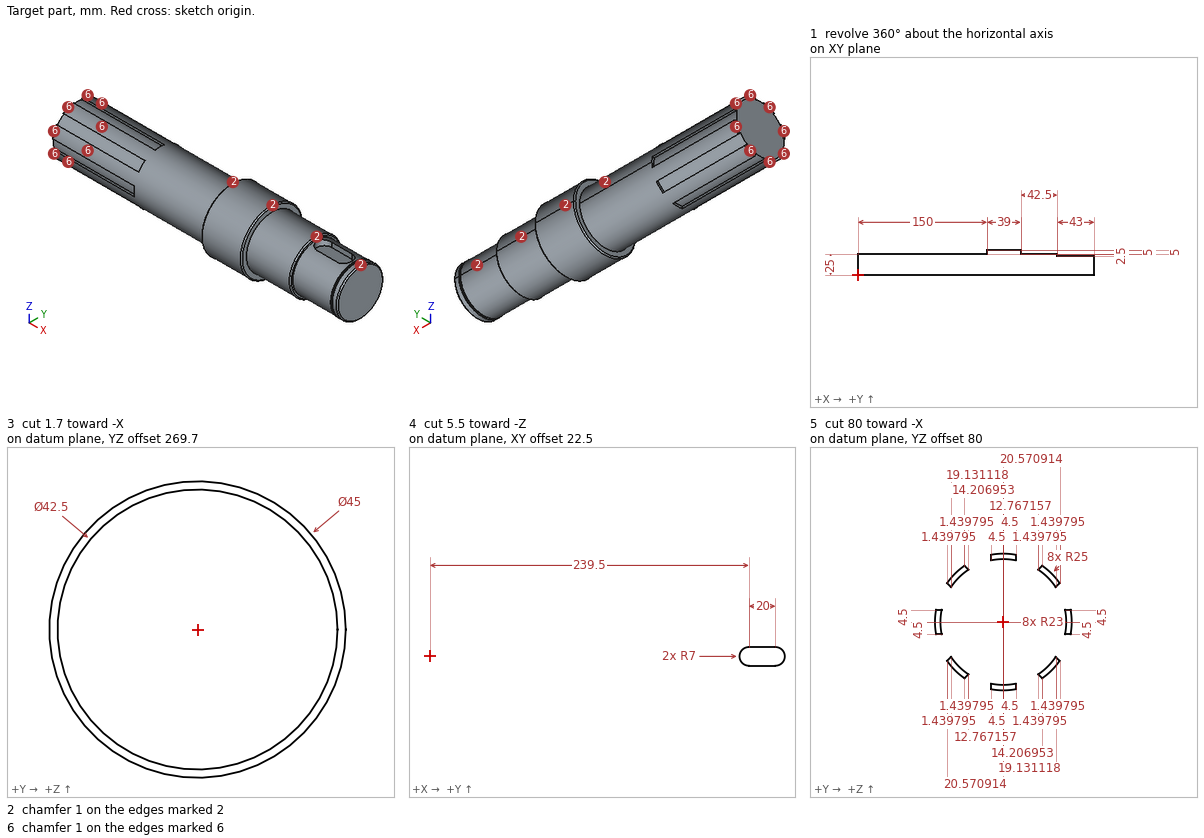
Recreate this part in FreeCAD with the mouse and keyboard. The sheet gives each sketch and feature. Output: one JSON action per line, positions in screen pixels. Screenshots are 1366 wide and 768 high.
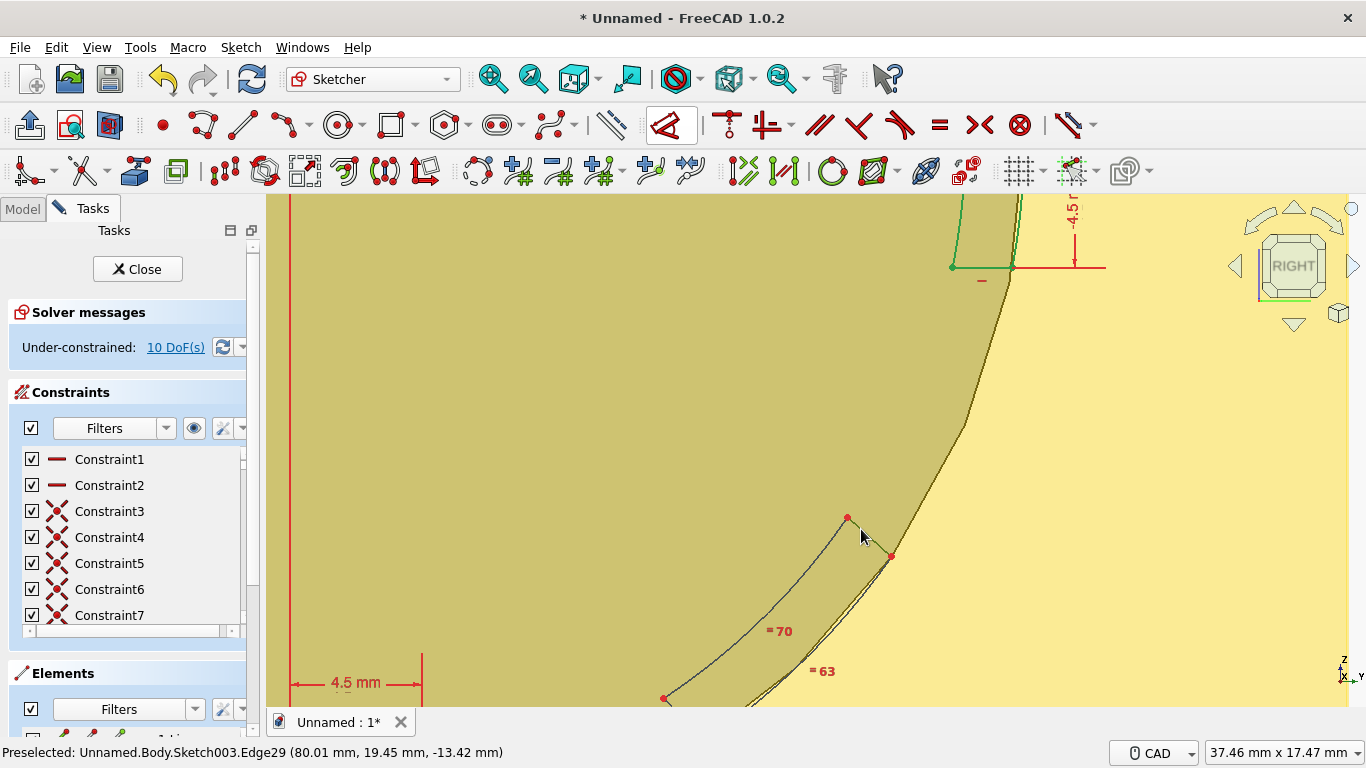
{"action": "left_click", "coordinate": [692, 126]}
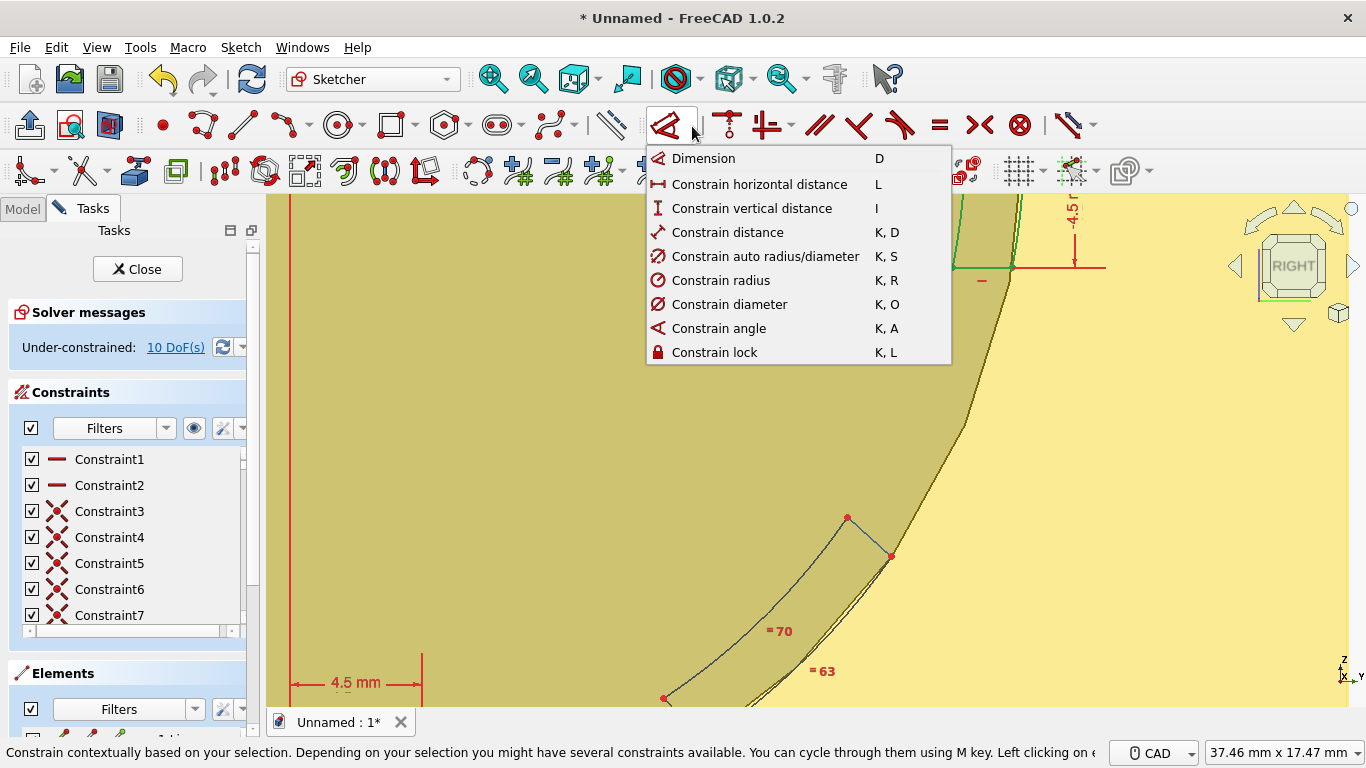
{"action": "left_click", "coordinate": [799, 184]}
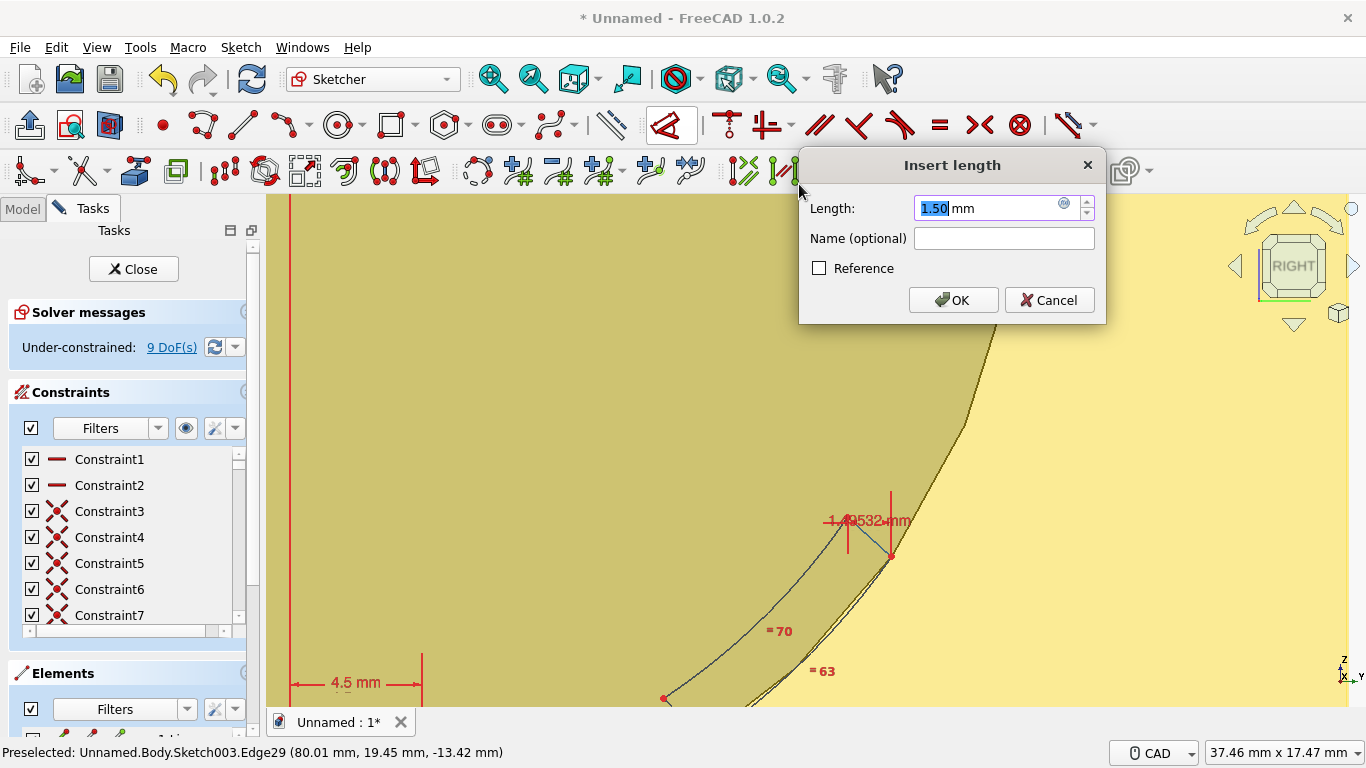
{"action": "type", "text": "1.439795"}
{"action": "key", "text": "Return"}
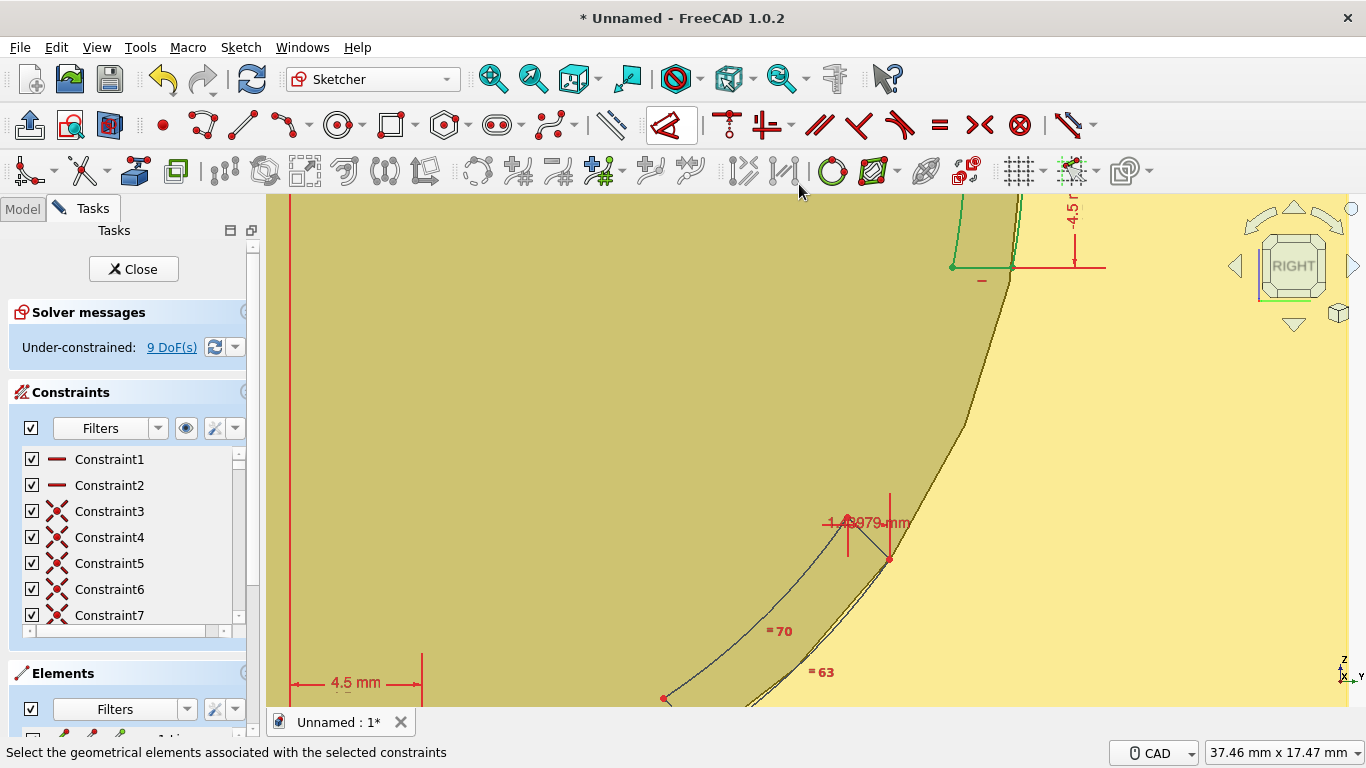
{"action": "scroll", "coordinate": [863, 530], "scroll_direction": "down", "scroll_amount": 8}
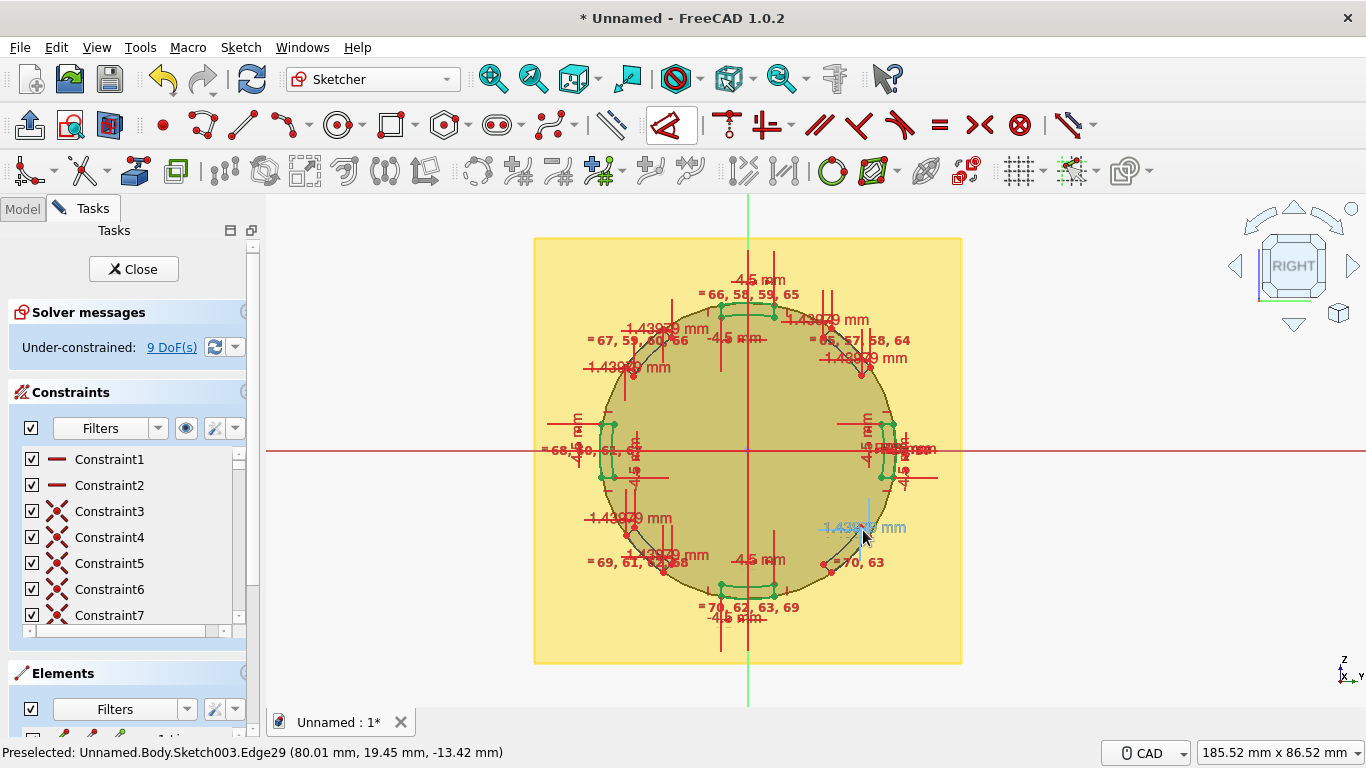
{"action": "scroll", "coordinate": [829, 570], "scroll_direction": "up", "scroll_amount": 8}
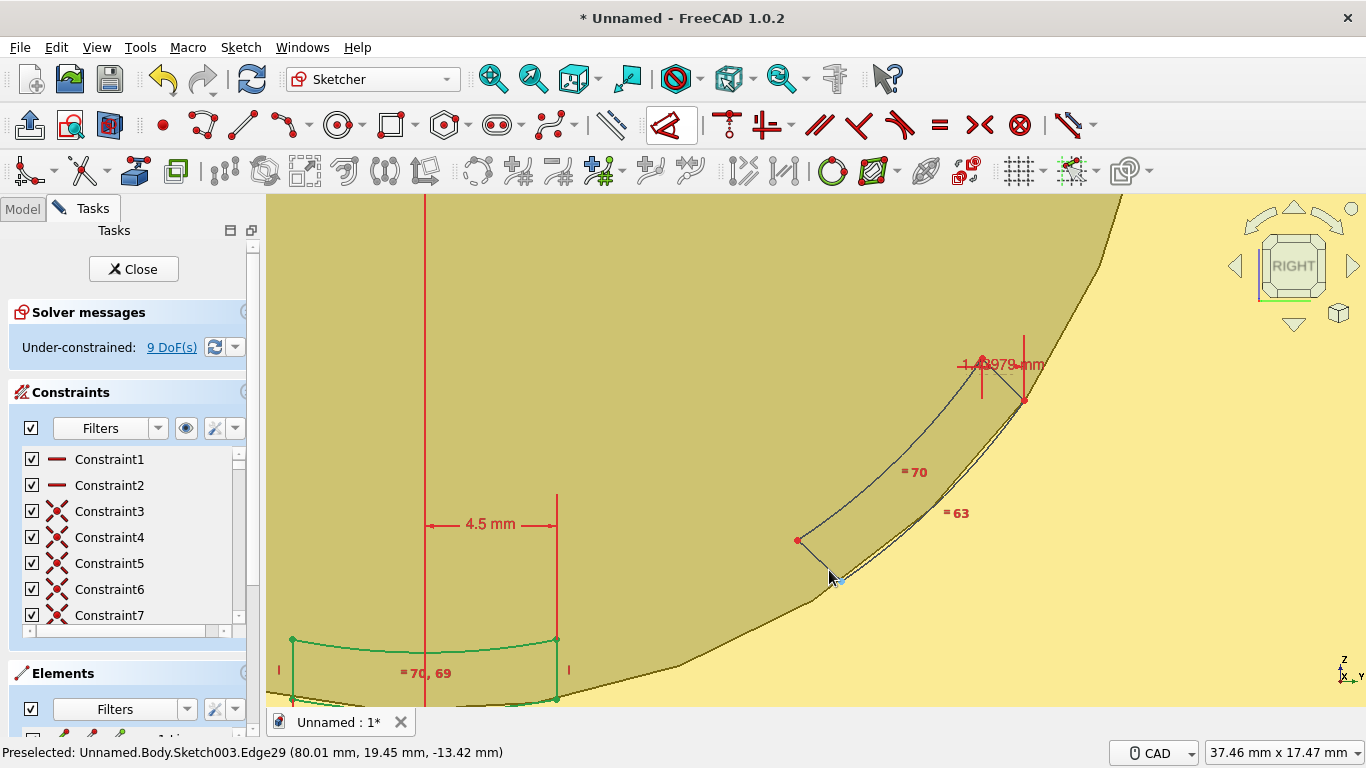
{"action": "left_click", "coordinate": [829, 569]}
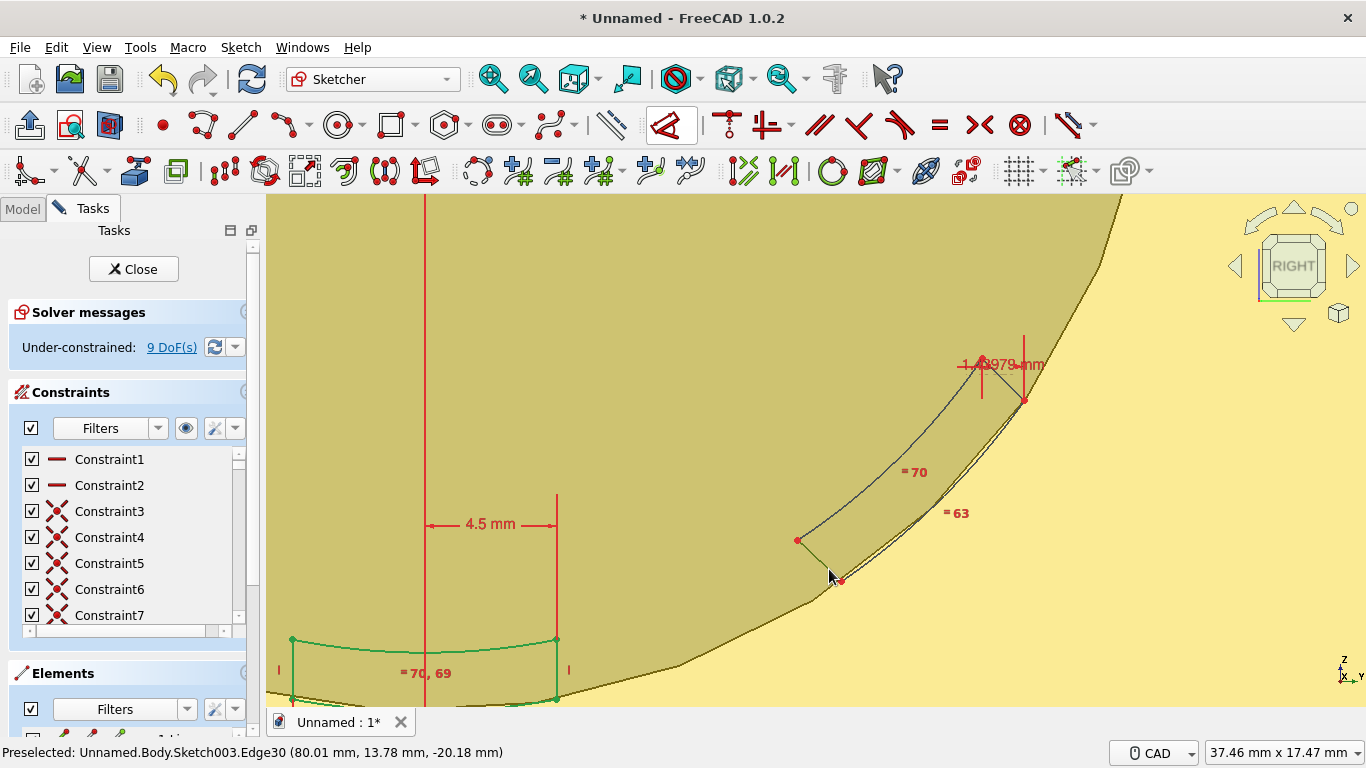
{"action": "left_click", "coordinate": [692, 126]}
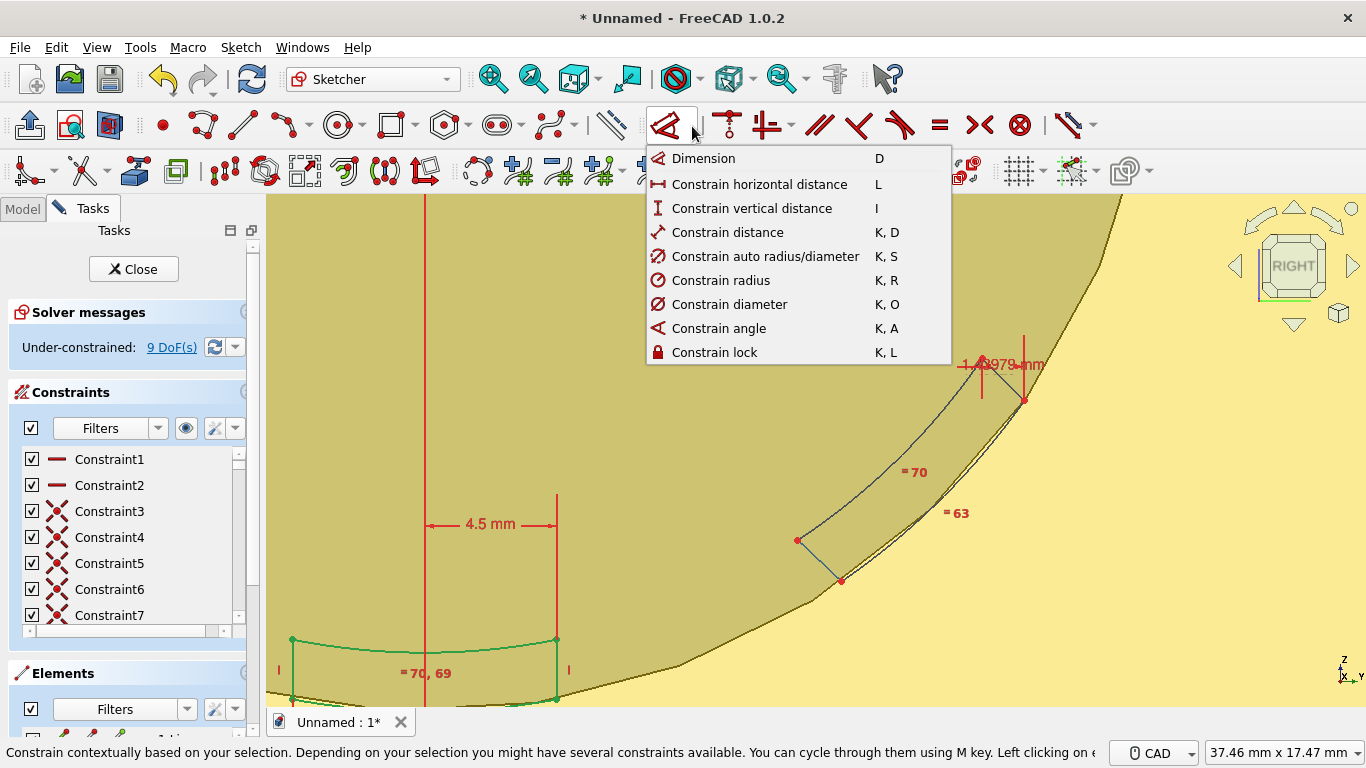
{"action": "left_click", "coordinate": [799, 184]}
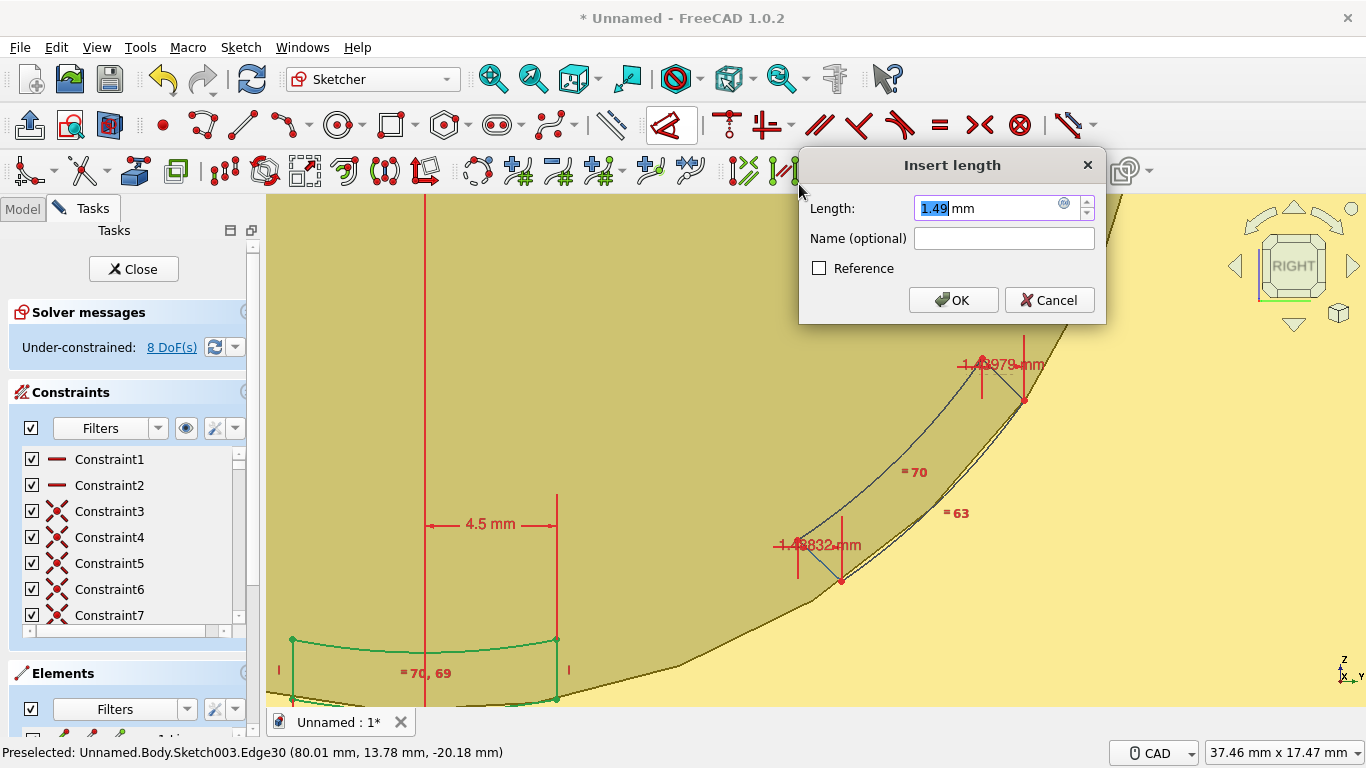
{"action": "type", "text": "1.439795"}
{"action": "key", "text": "Return"}